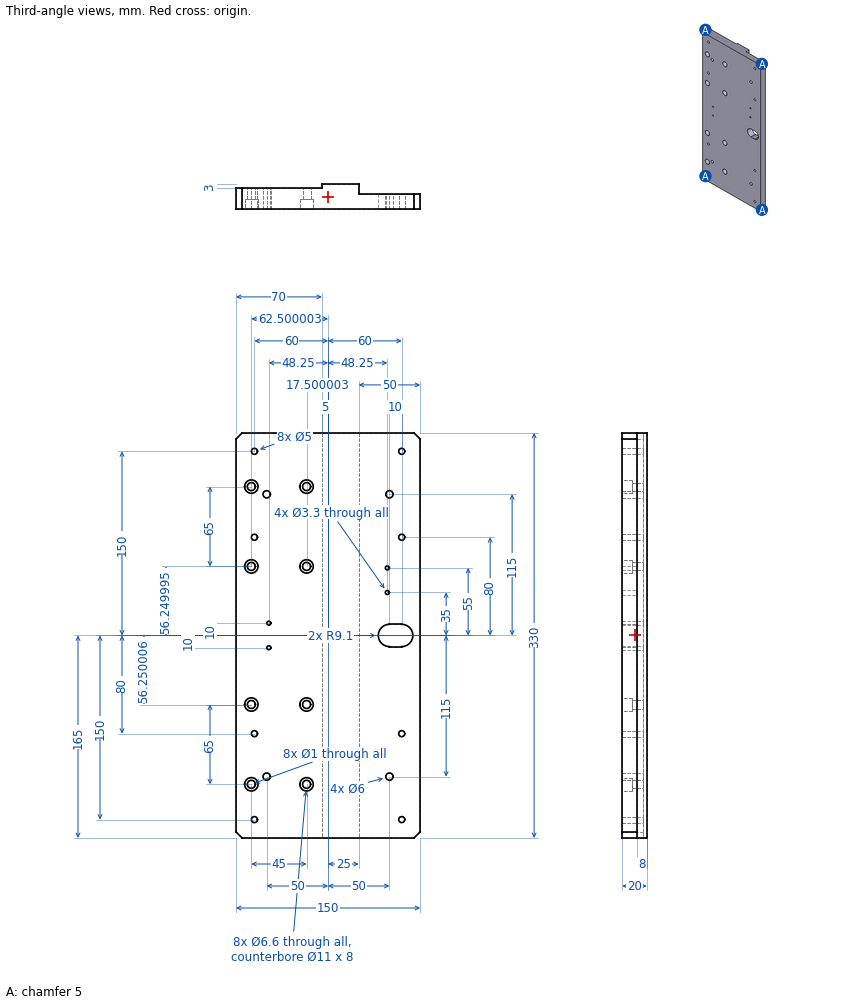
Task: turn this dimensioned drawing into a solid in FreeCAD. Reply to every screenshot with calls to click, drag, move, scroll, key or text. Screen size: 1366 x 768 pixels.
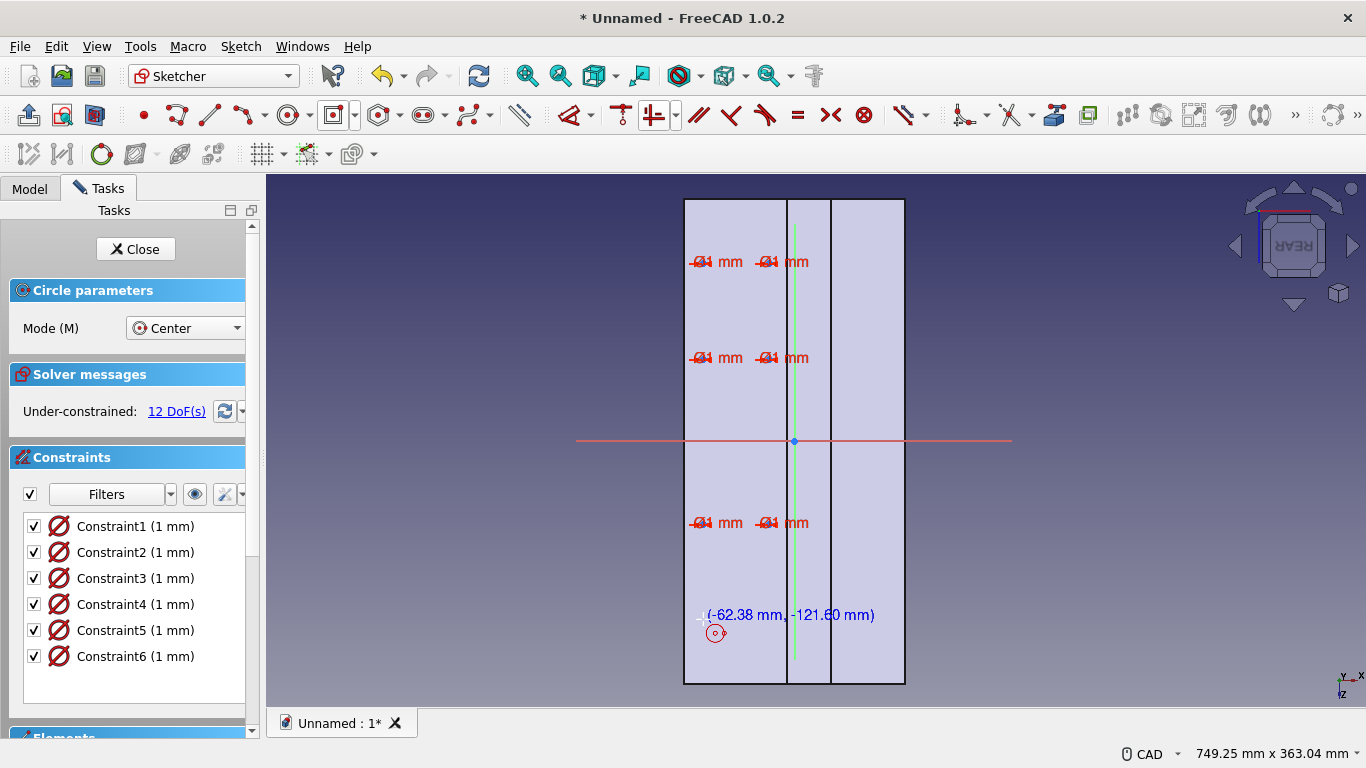
click(703, 619)
move(703, 619)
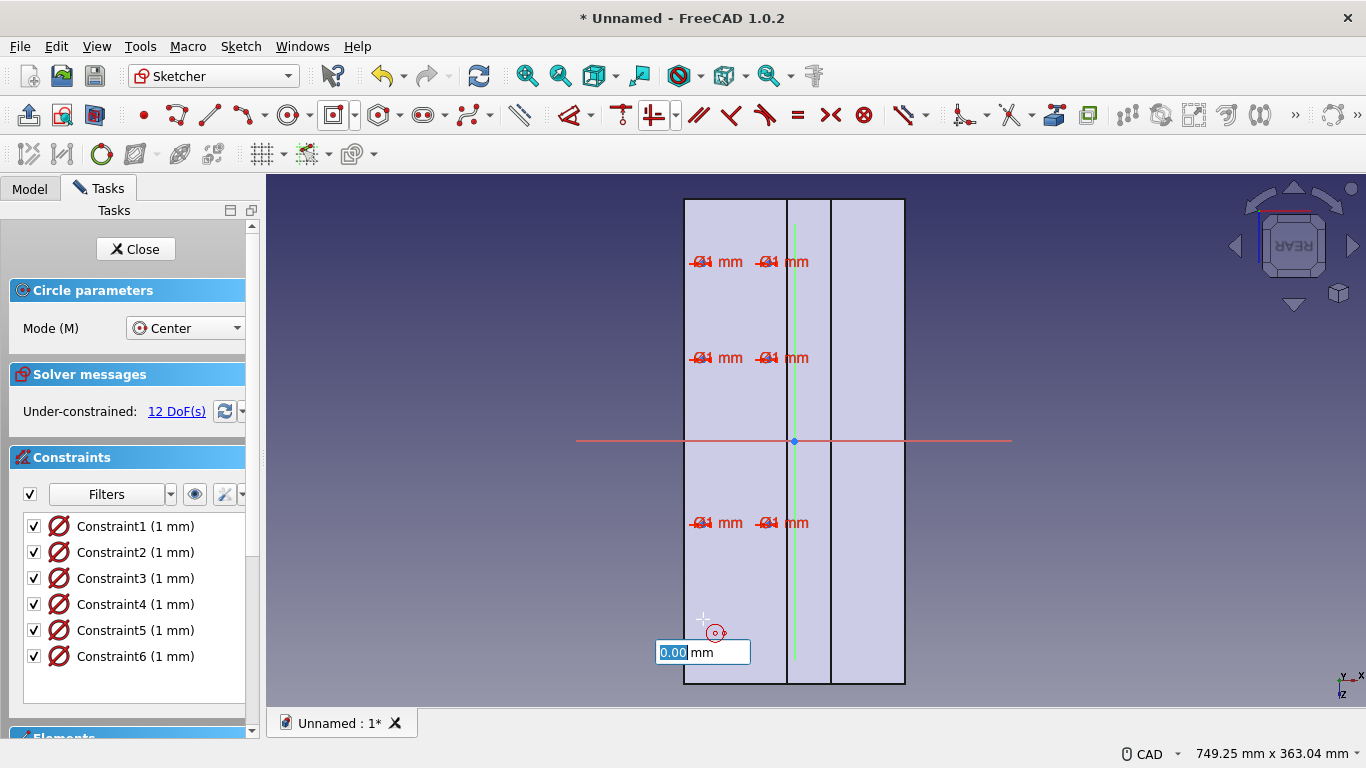
text(1)
key(Return)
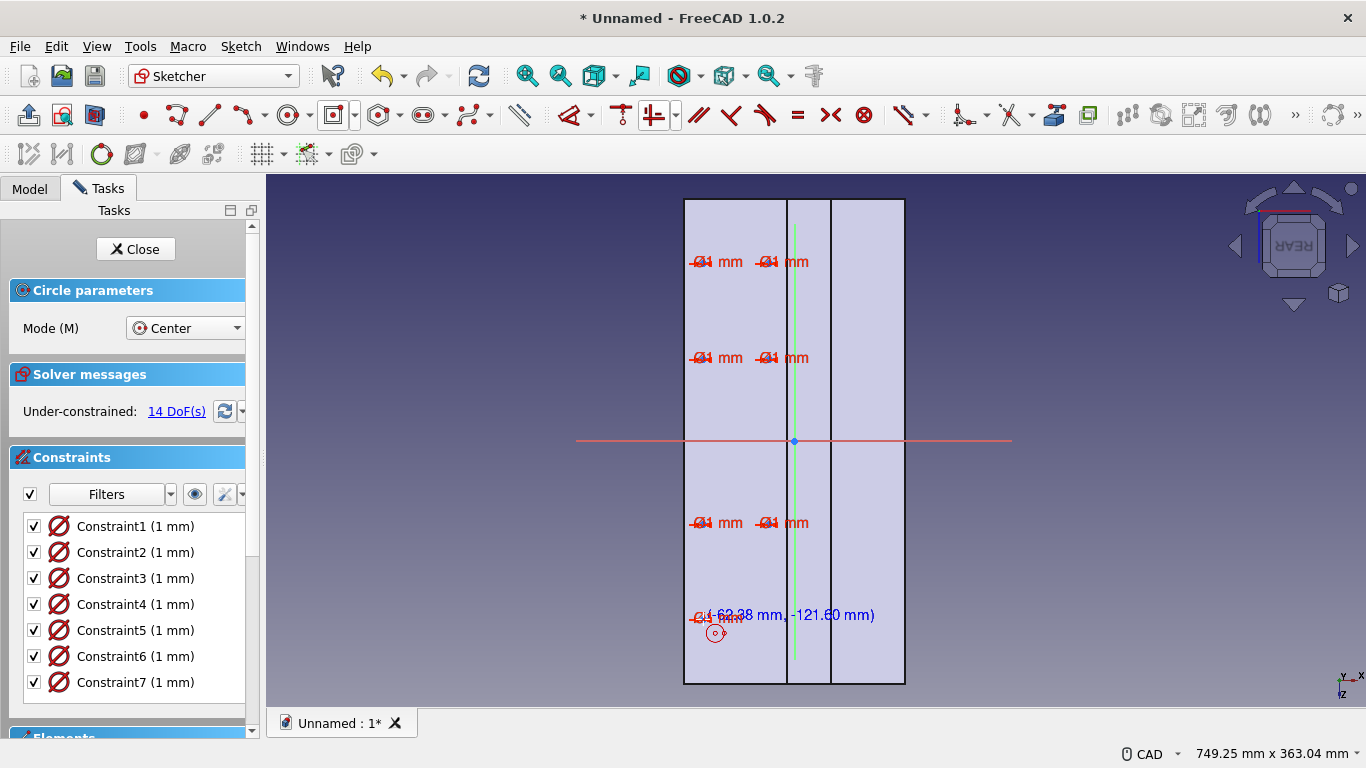
scroll(769, 619, up, 18)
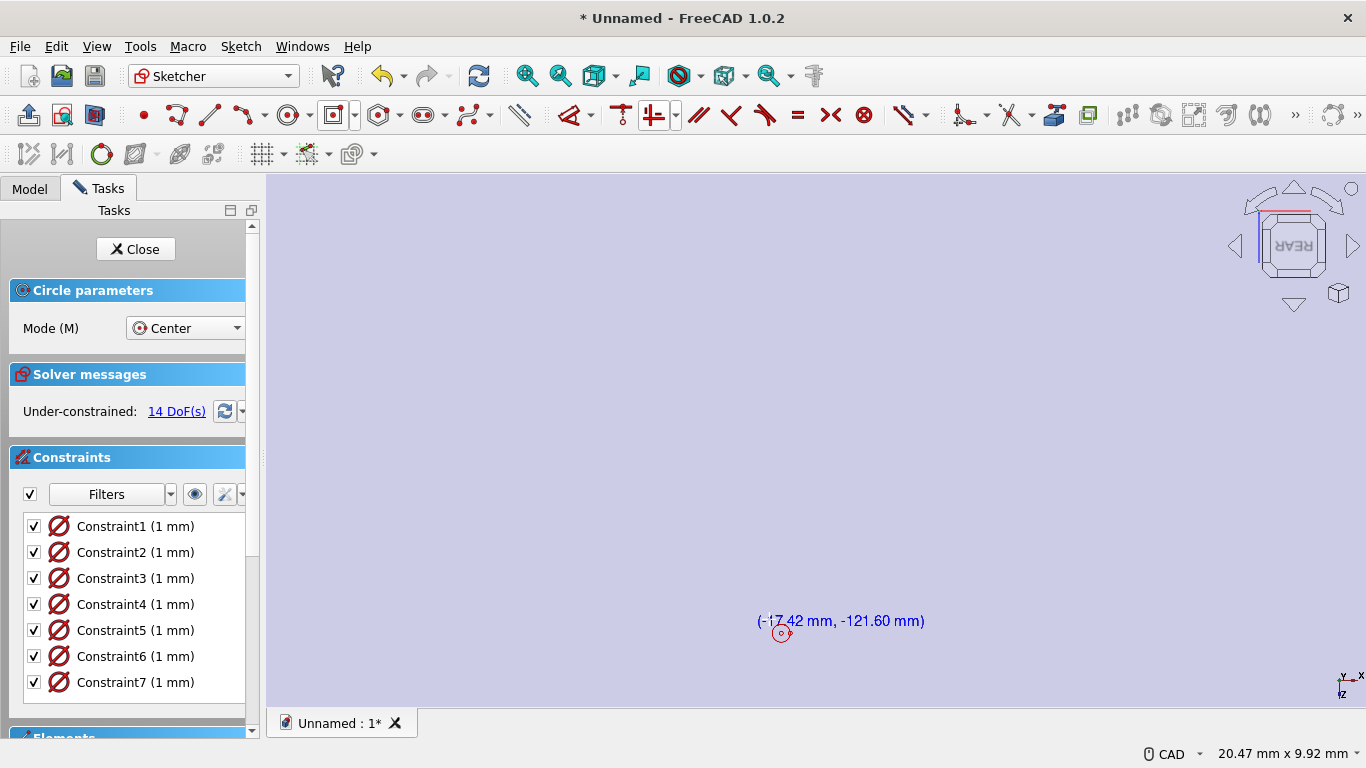
scroll(769, 619, down, 18)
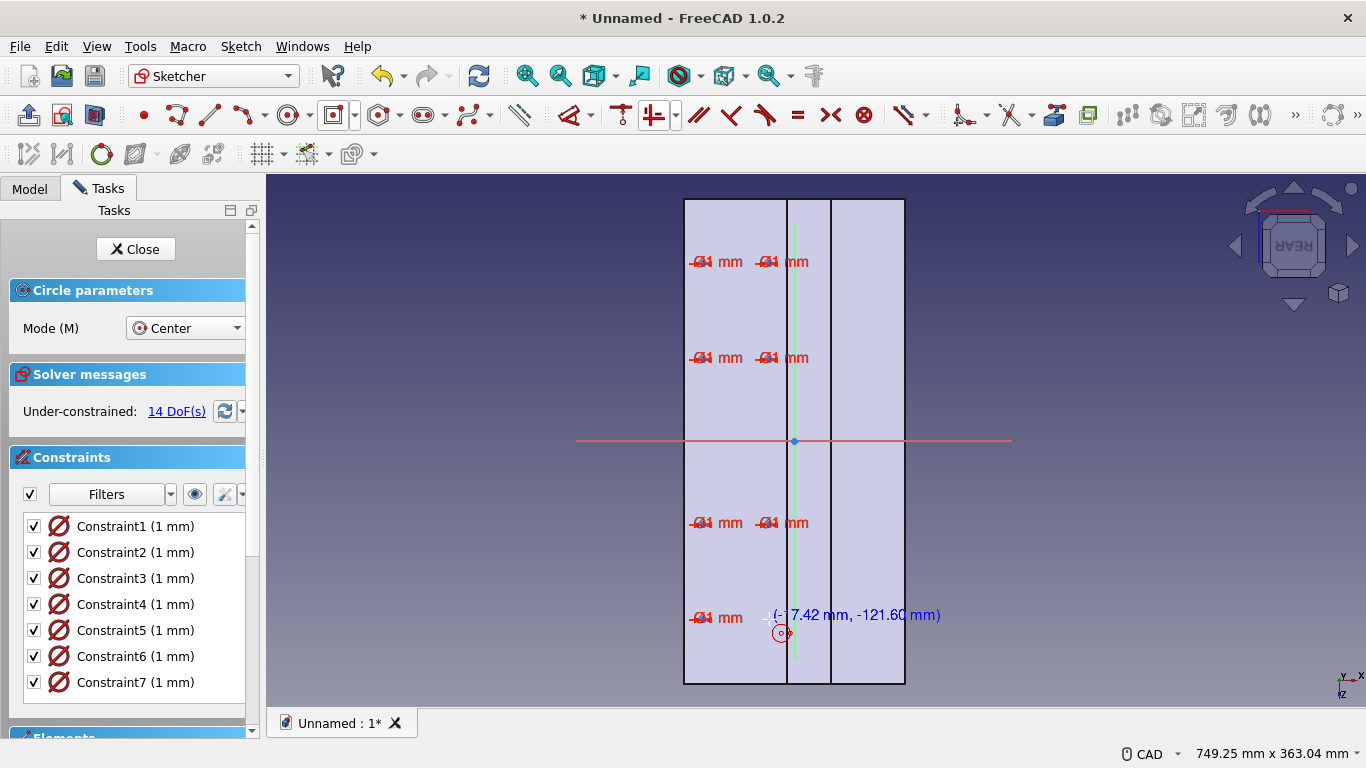
click(769, 619)
move(769, 619)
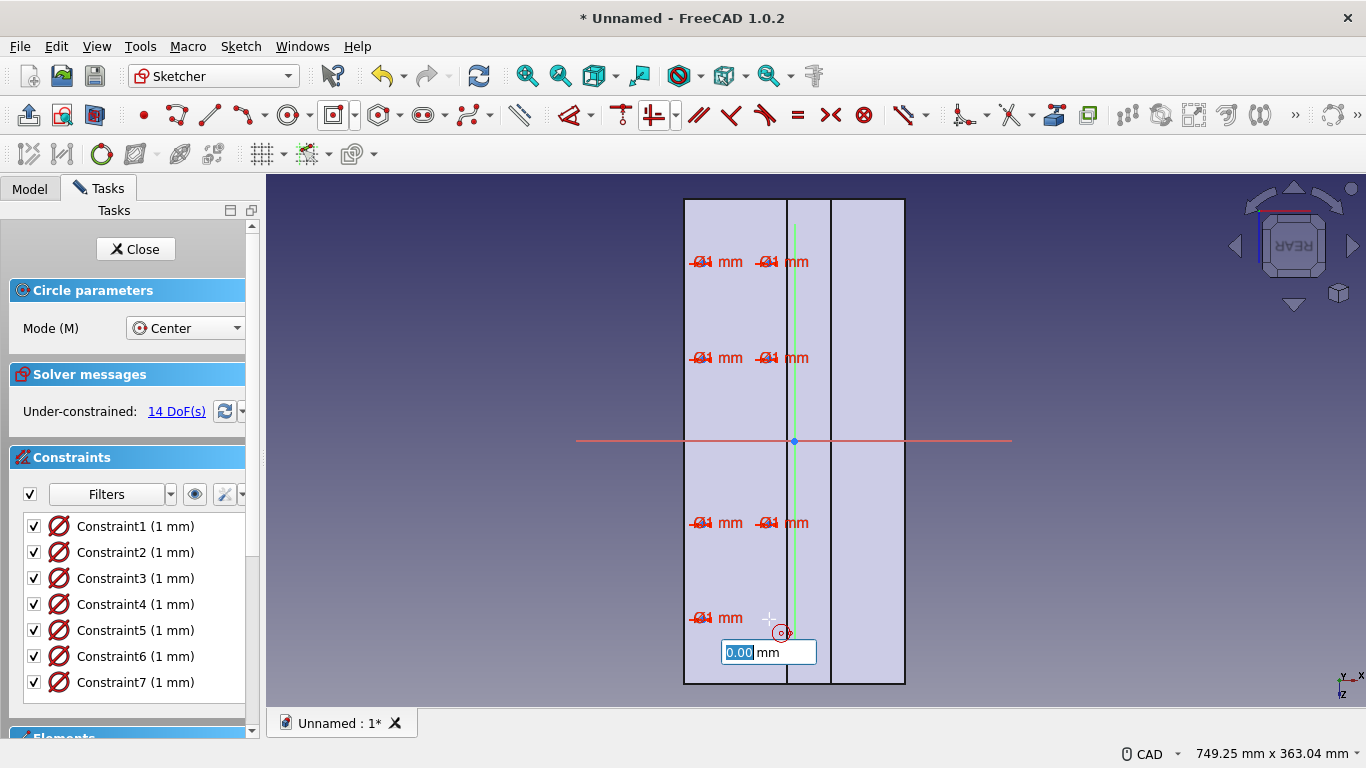
text(1)
key(Return)
key(Escape)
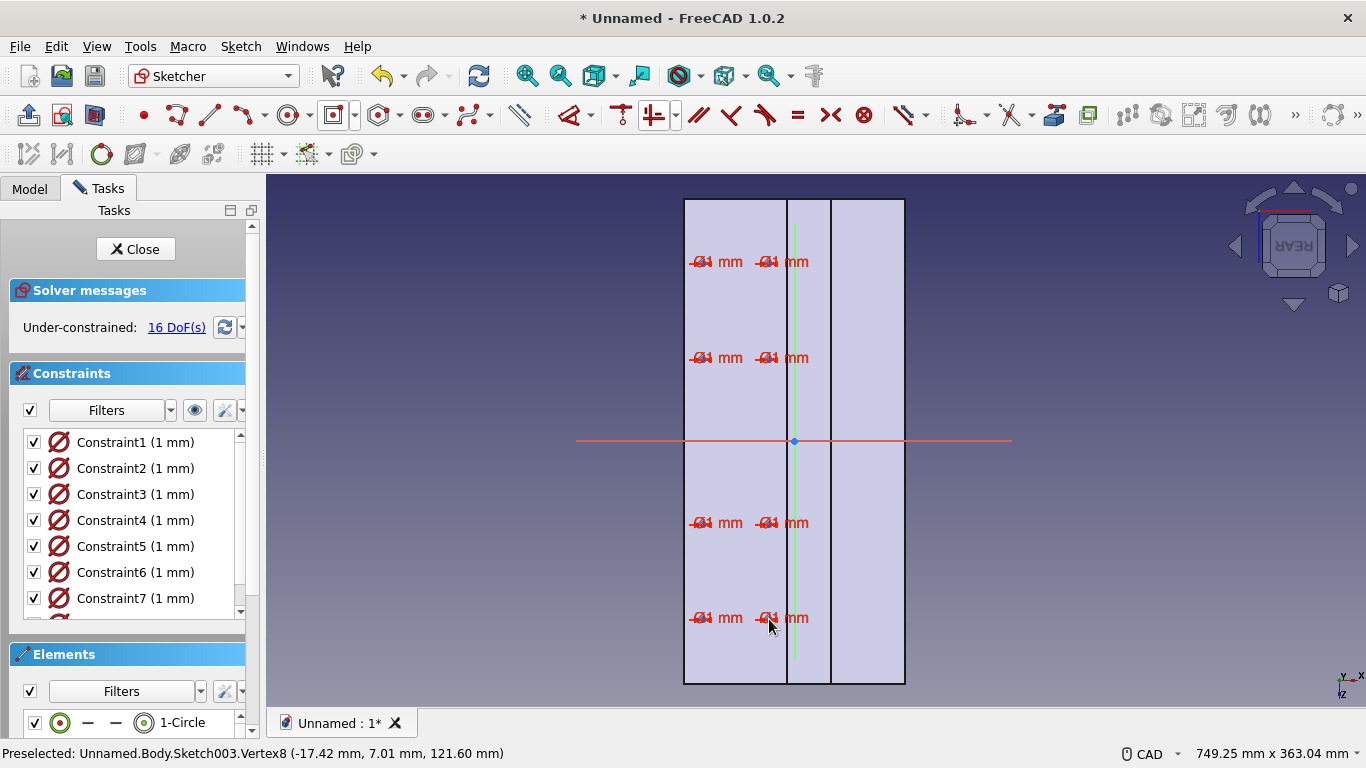
click(703, 264)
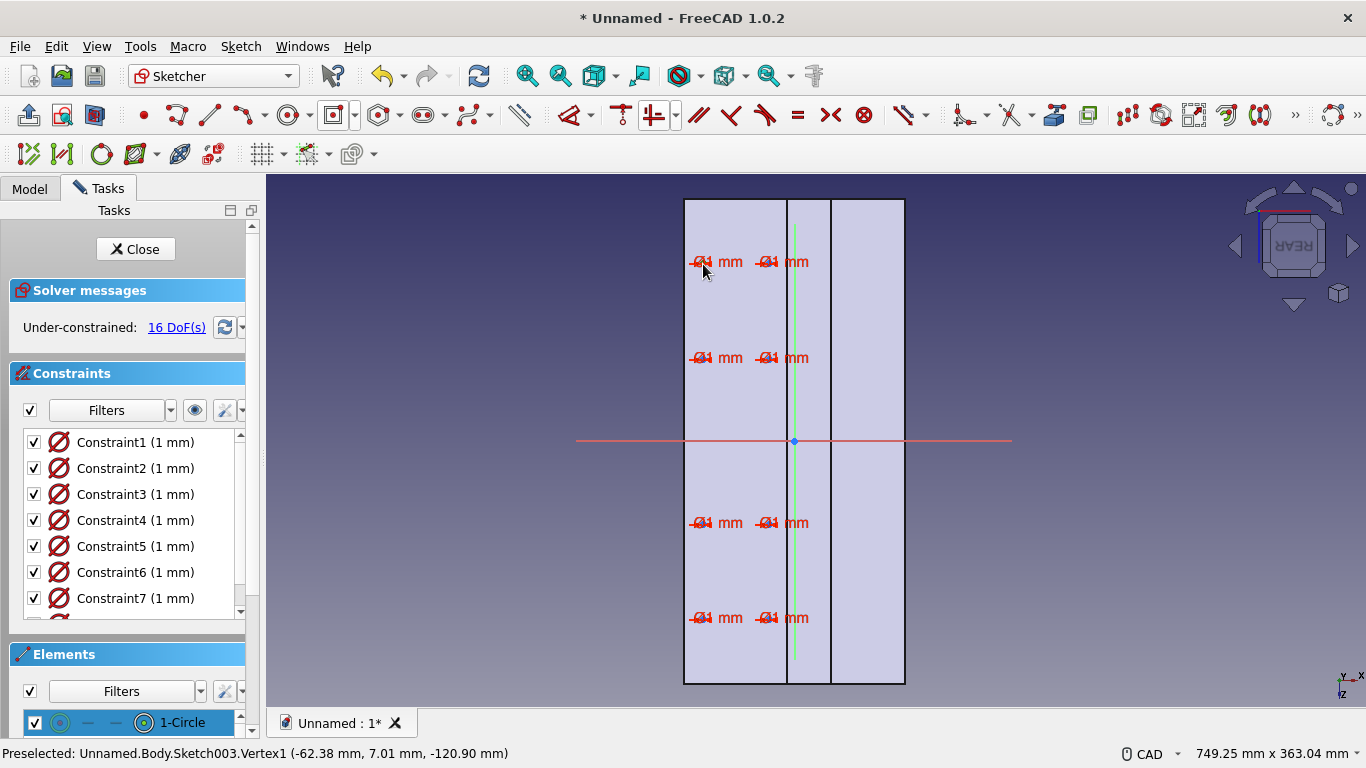
click(769, 264)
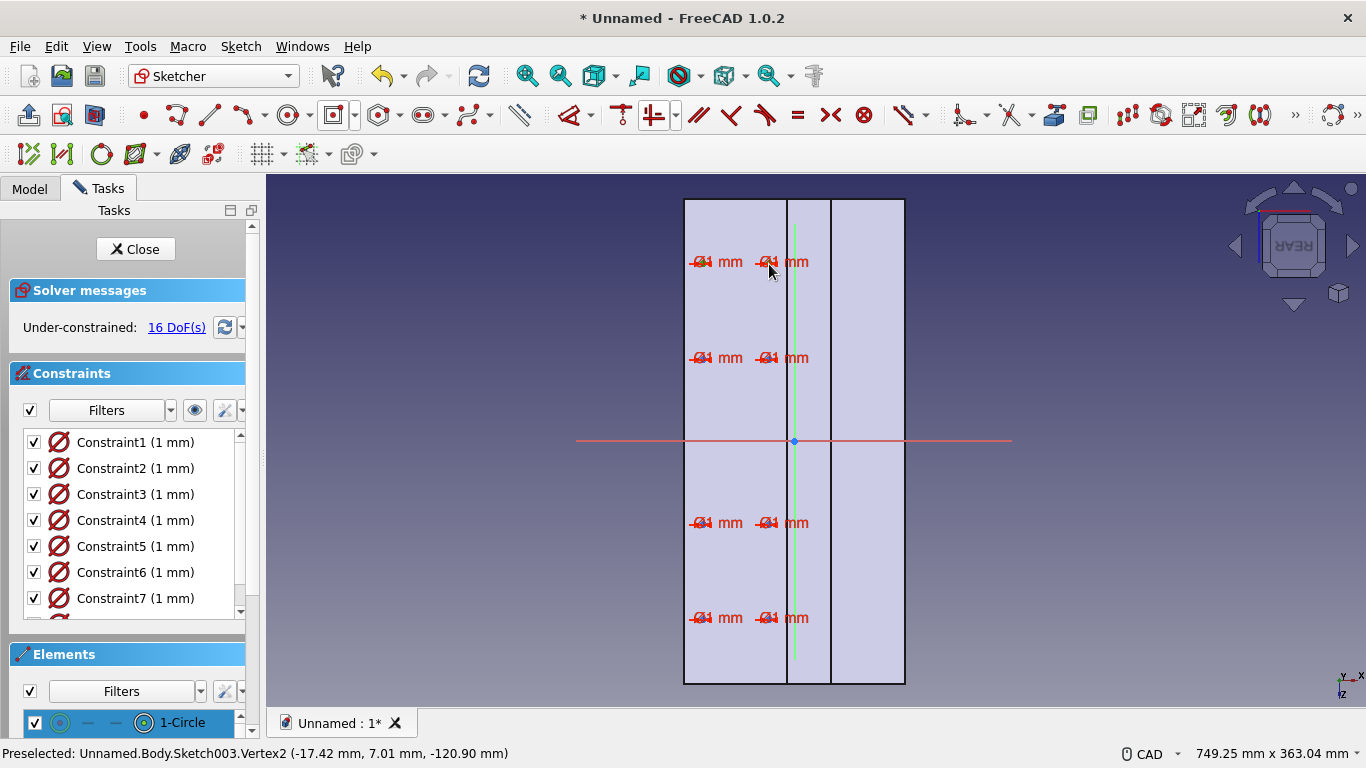
click(676, 116)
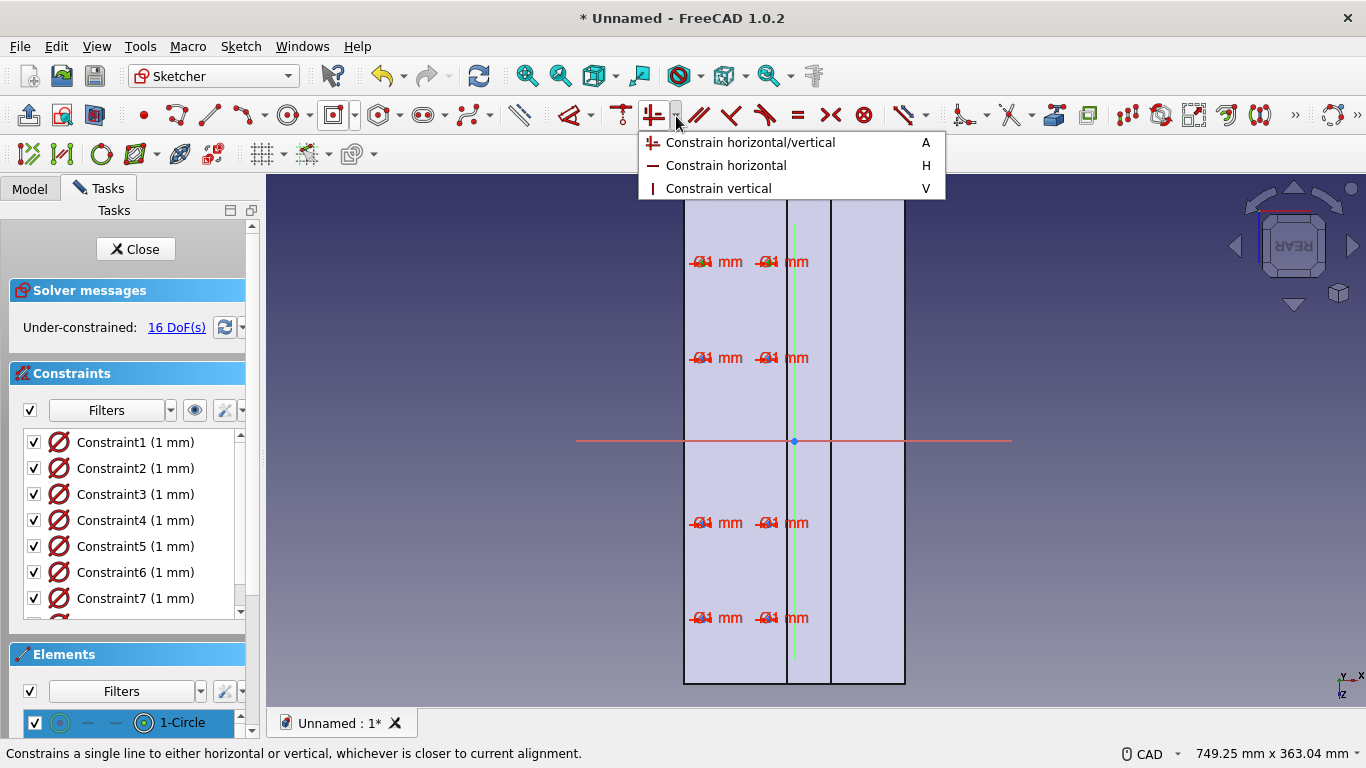
click(792, 166)